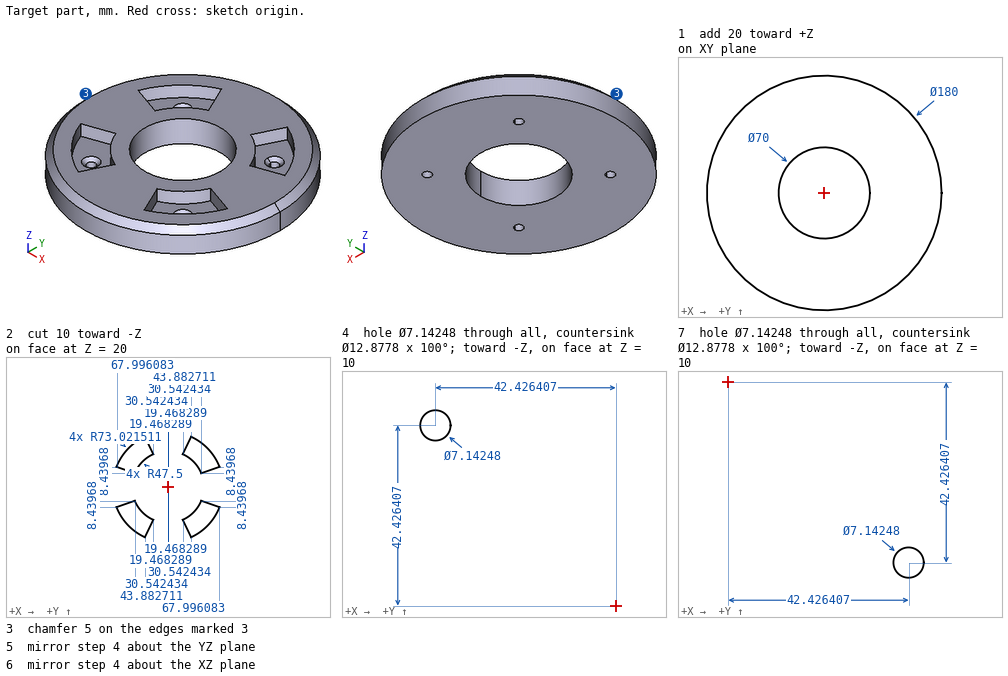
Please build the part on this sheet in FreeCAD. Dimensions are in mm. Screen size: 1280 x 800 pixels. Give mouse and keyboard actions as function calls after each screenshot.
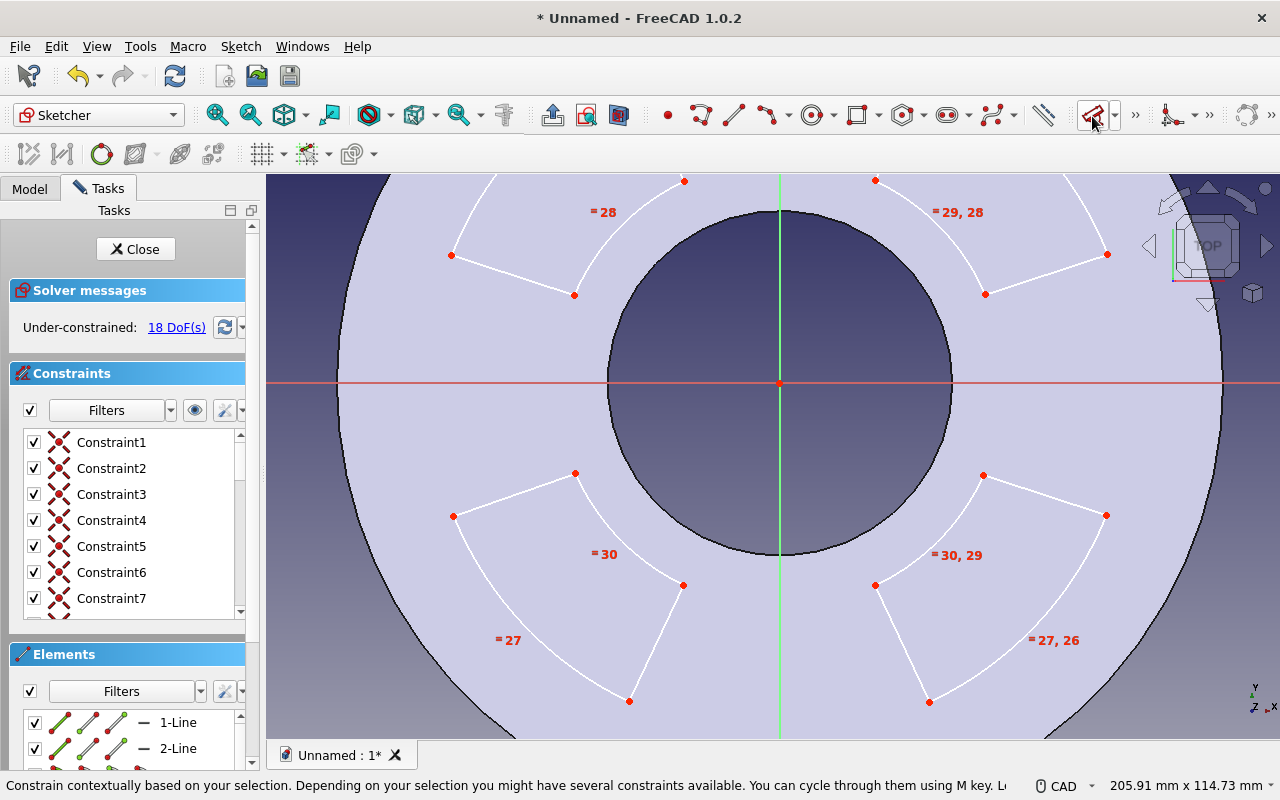
click(475, 207)
click(438, 559)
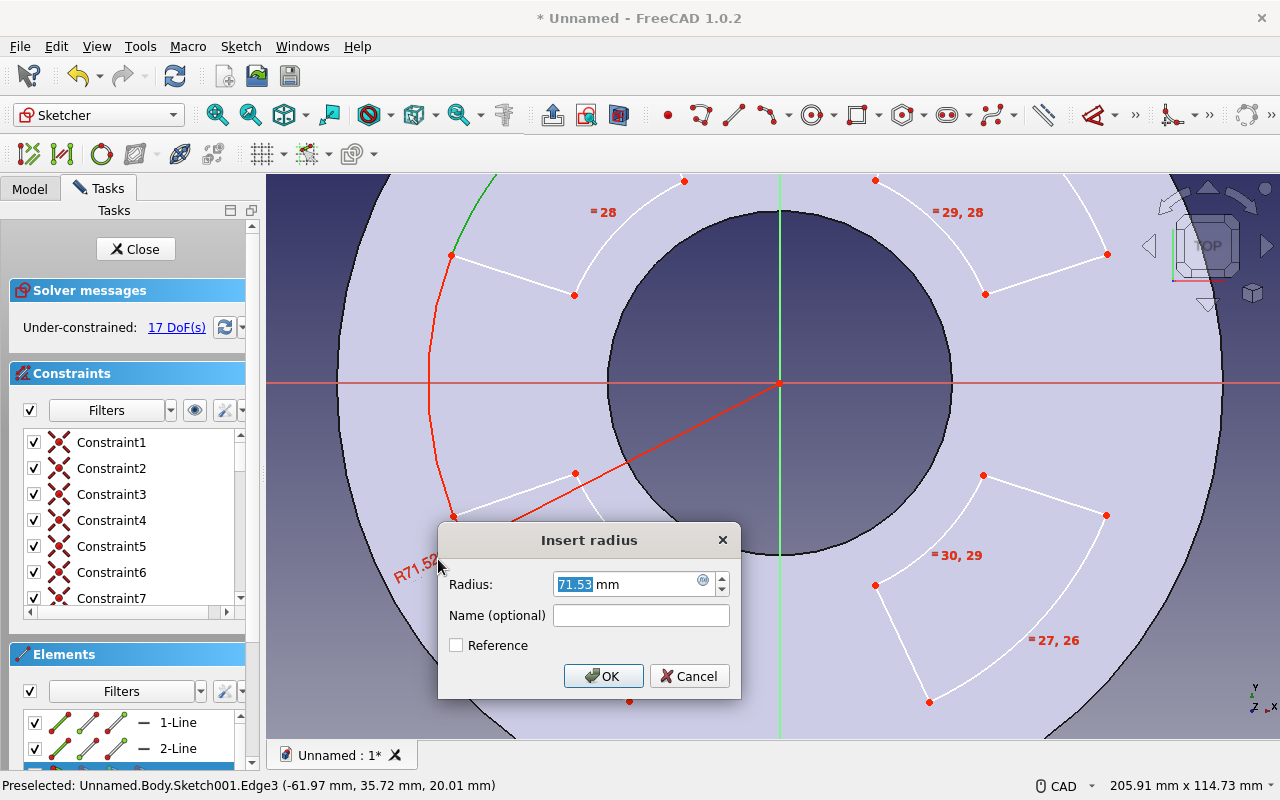
text(73.021511)
key(Return)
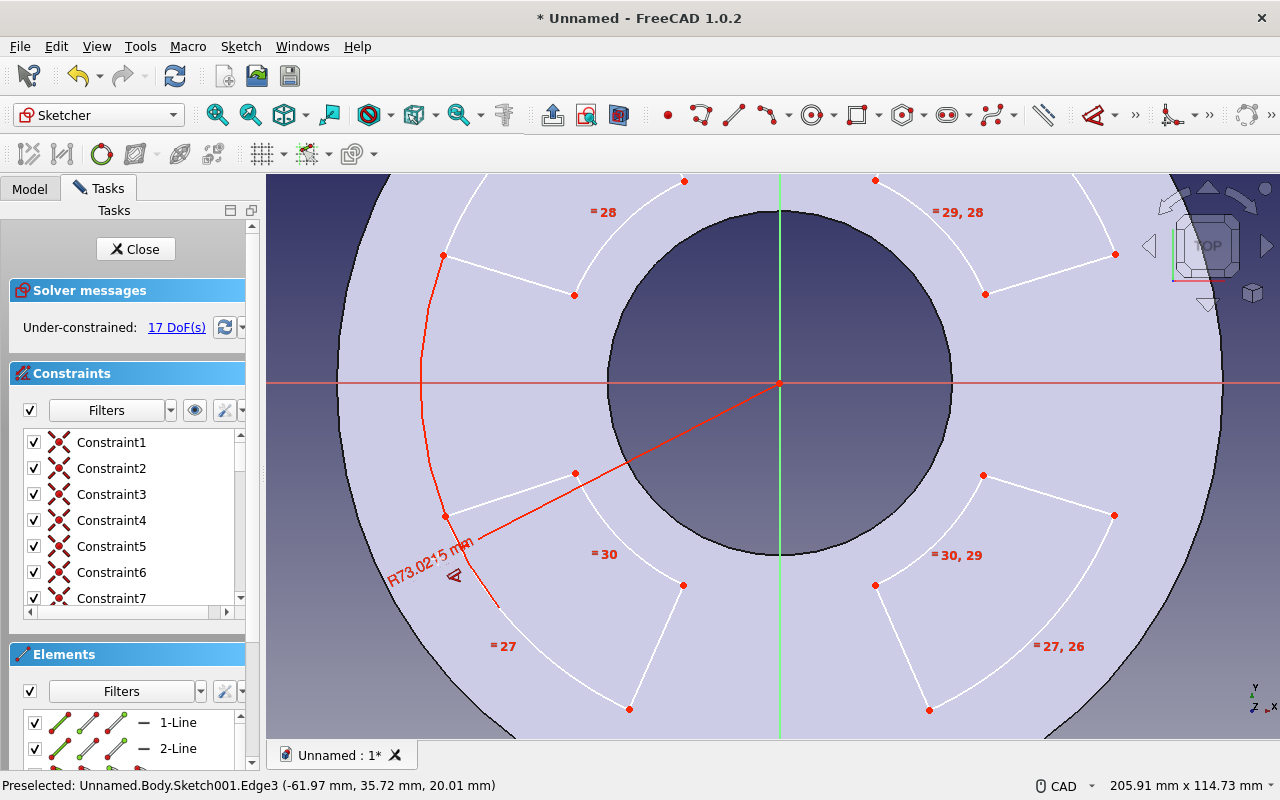
click(643, 207)
click(526, 406)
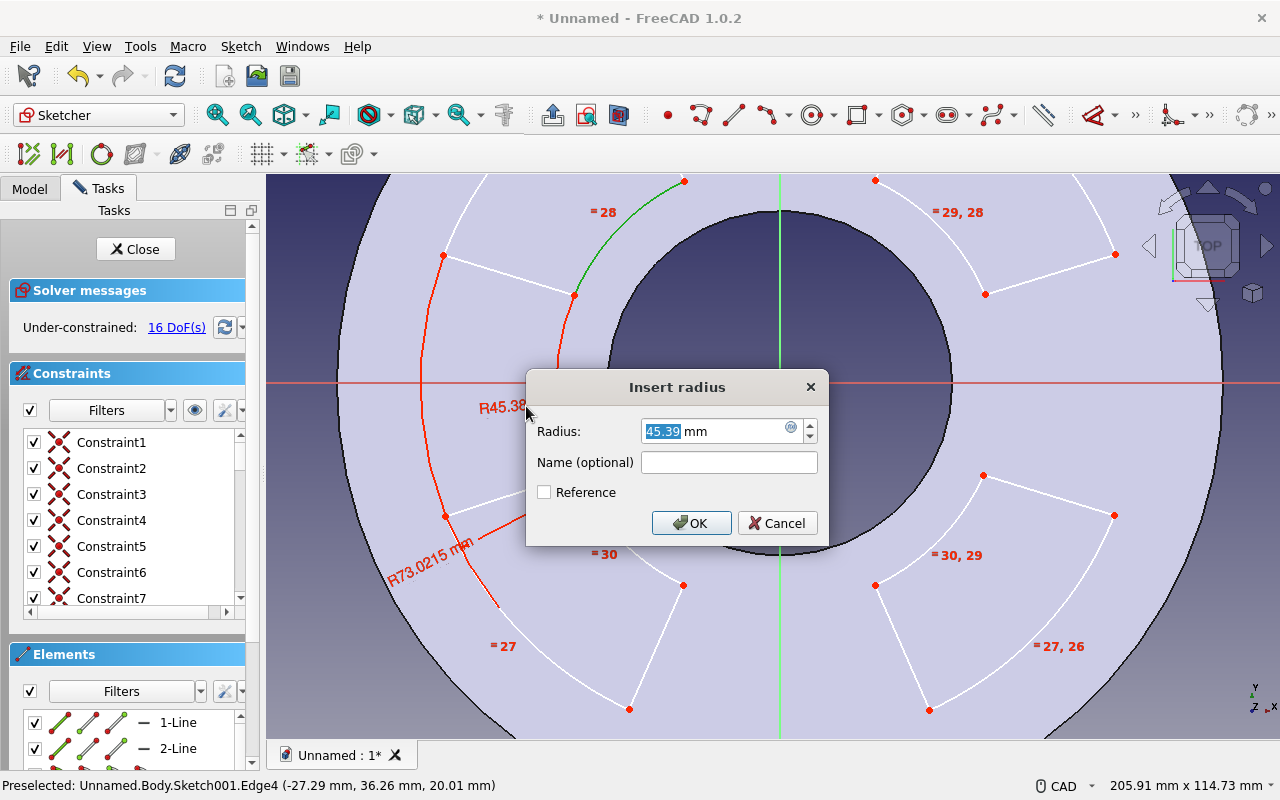
text(47.5)
key(Return)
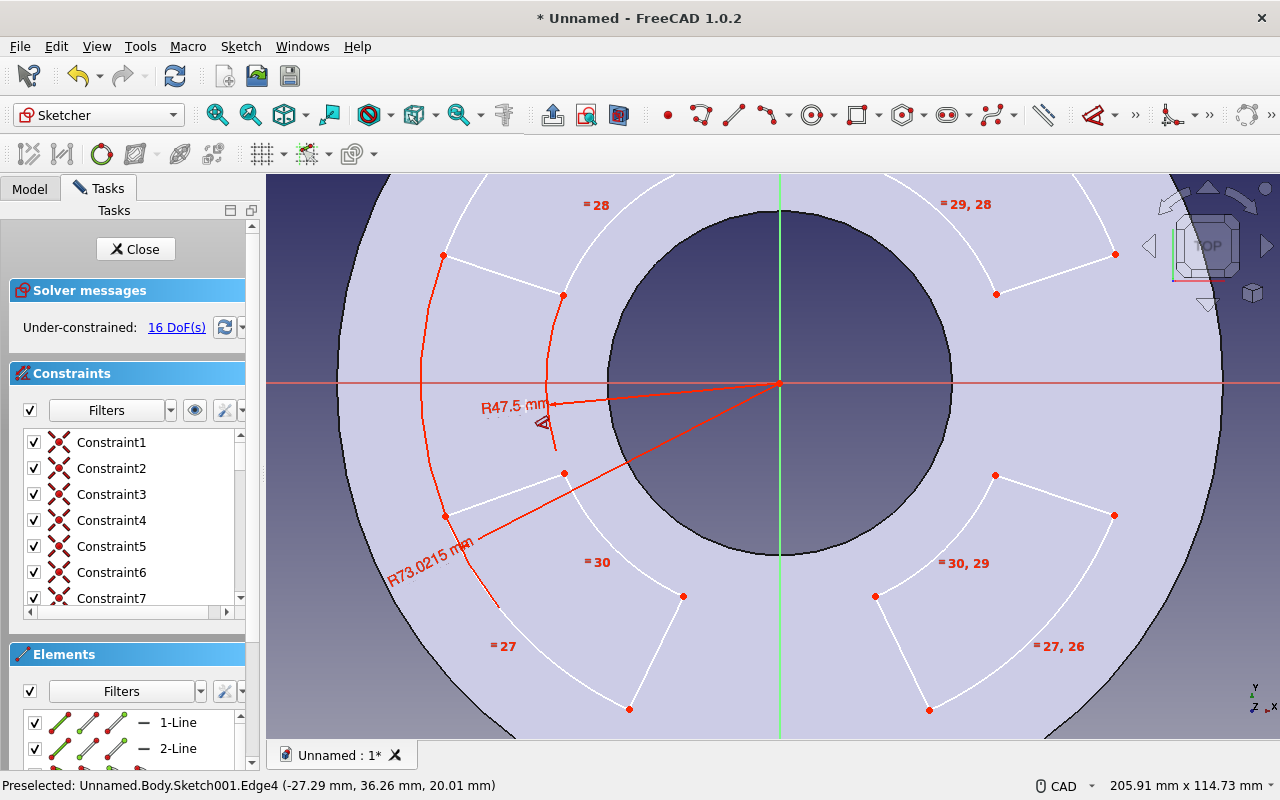
click(480, 267)
click(410, 275)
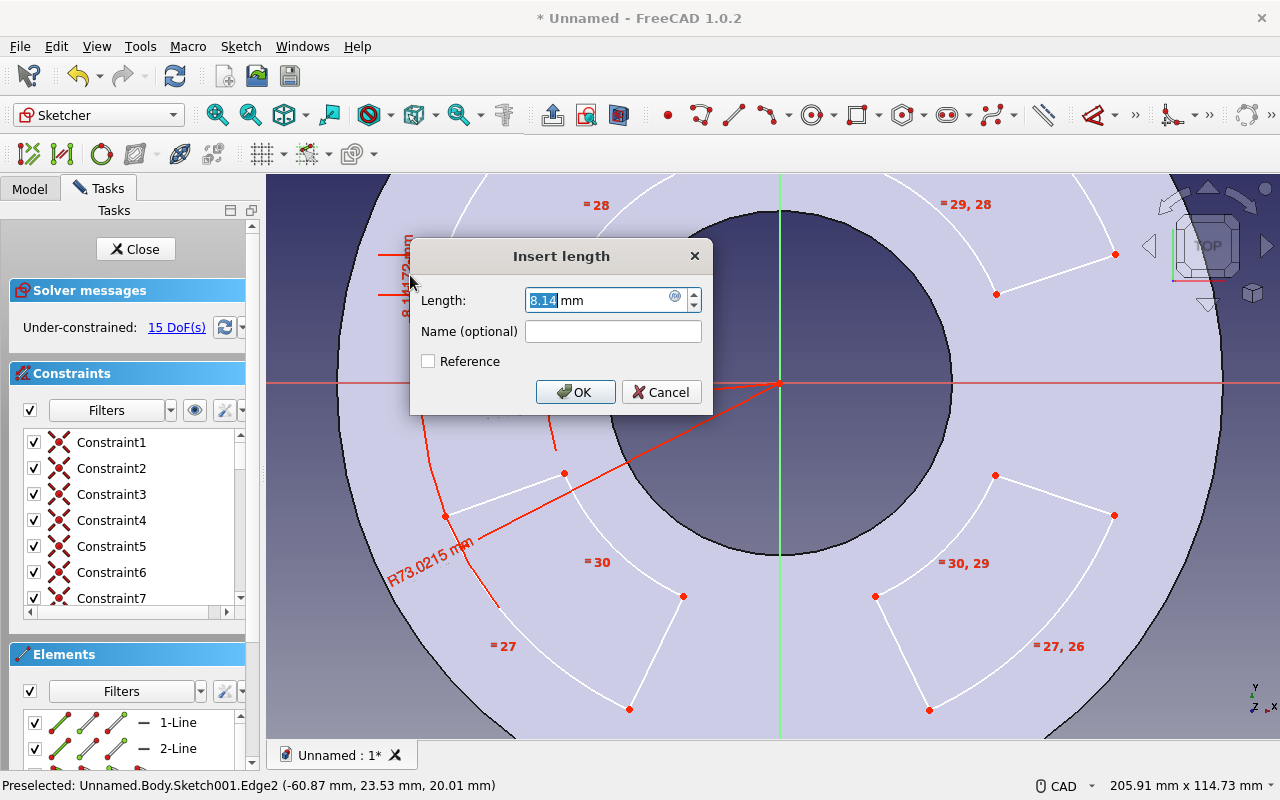
text(8.43968)
key(Return)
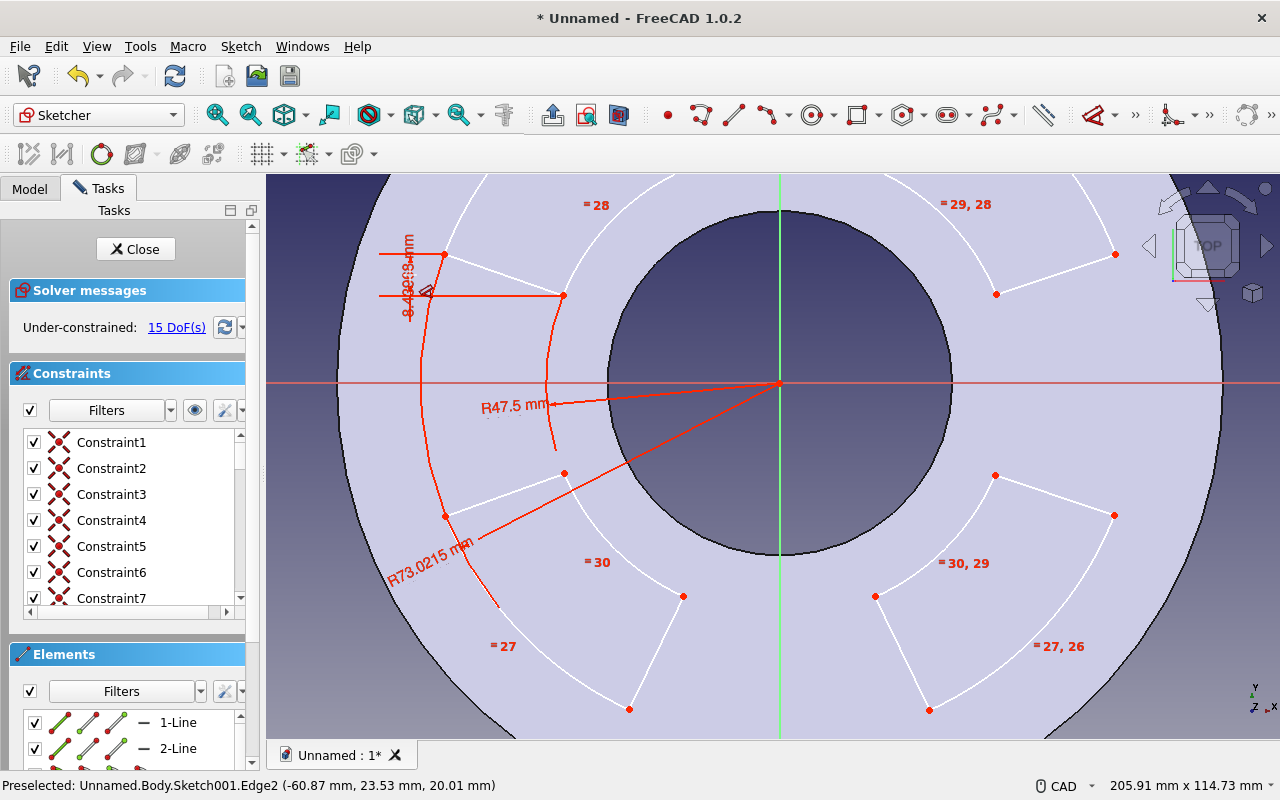
click(1032, 283)
click(963, 275)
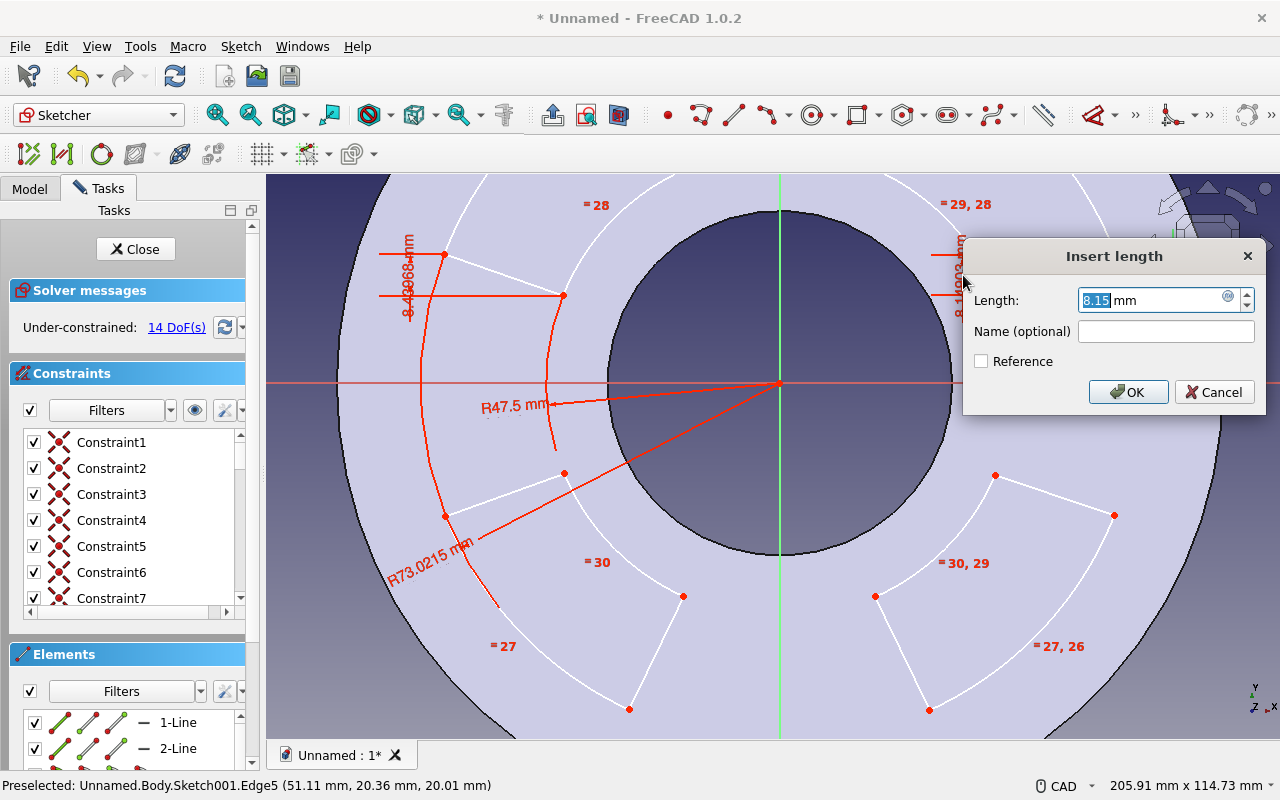
text(8.43968)
key(Return)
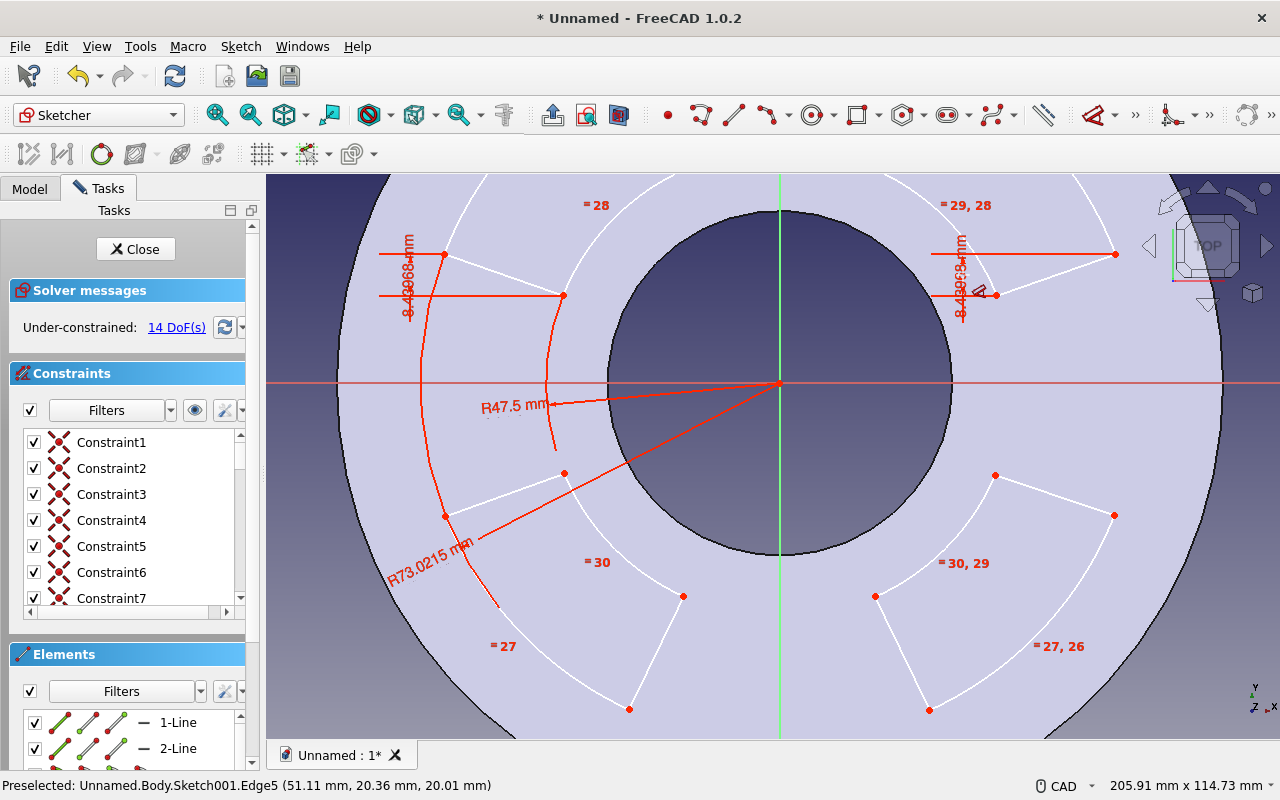
click(1079, 503)
click(961, 495)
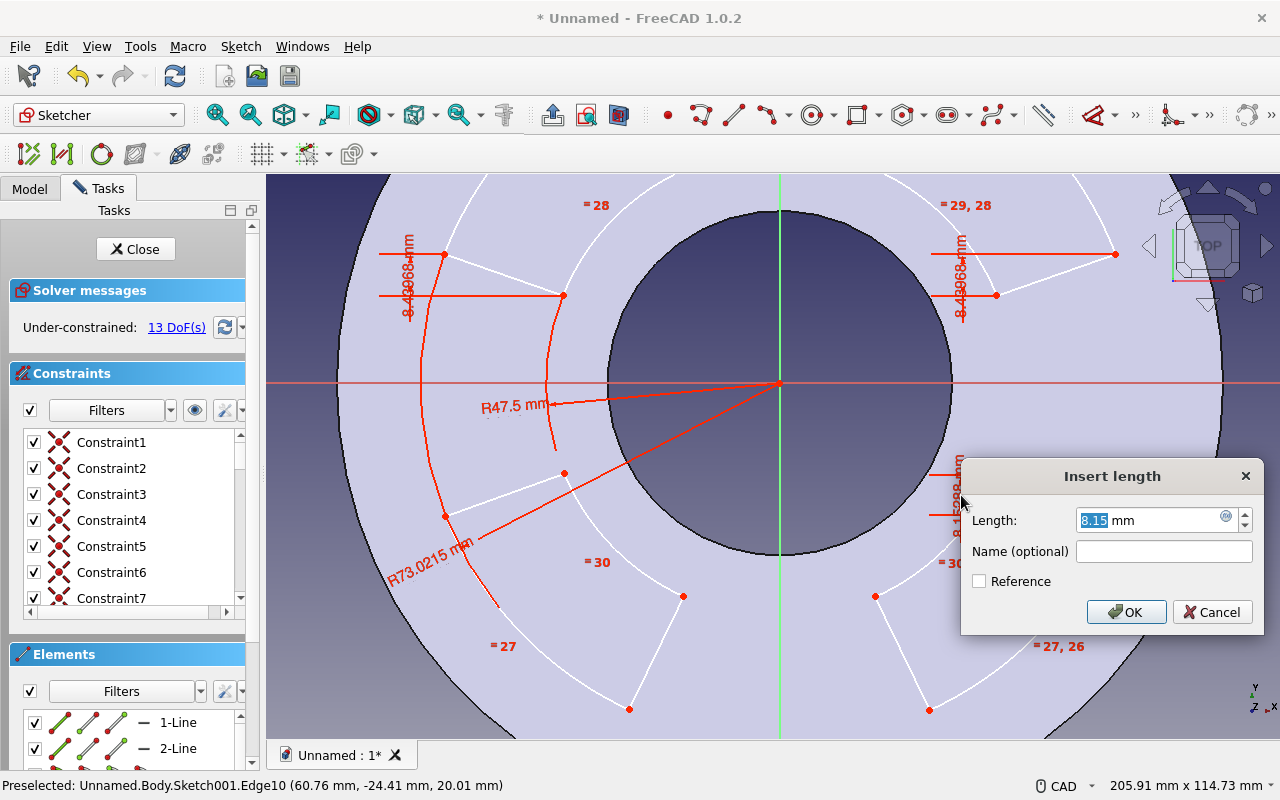
text(8.43968)
key(Return)